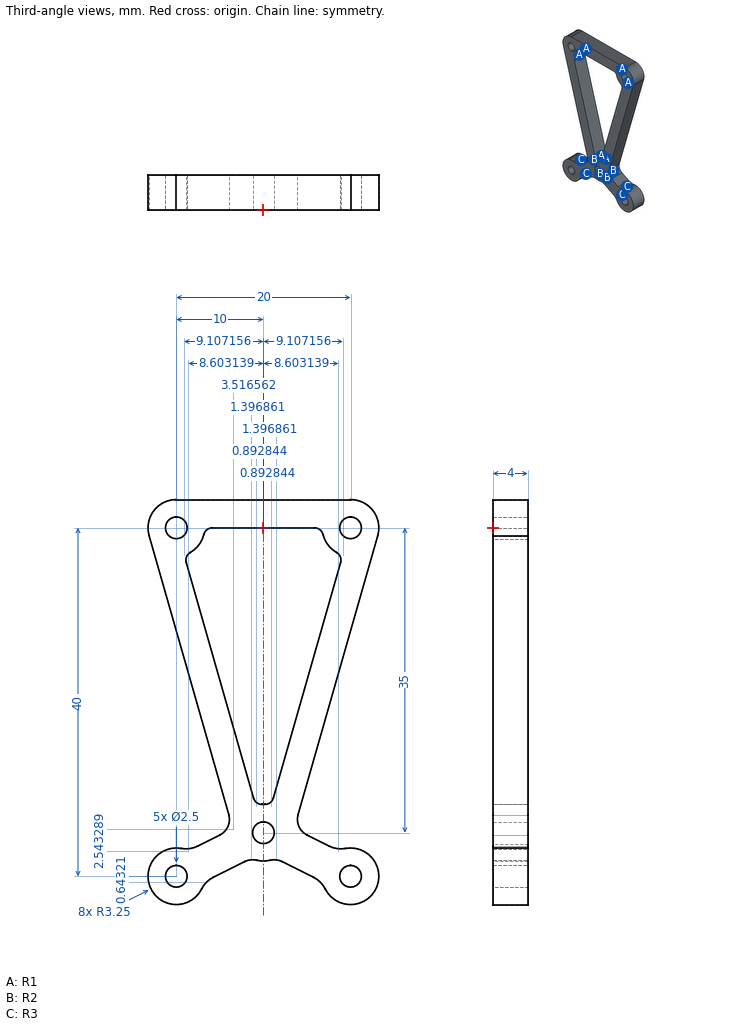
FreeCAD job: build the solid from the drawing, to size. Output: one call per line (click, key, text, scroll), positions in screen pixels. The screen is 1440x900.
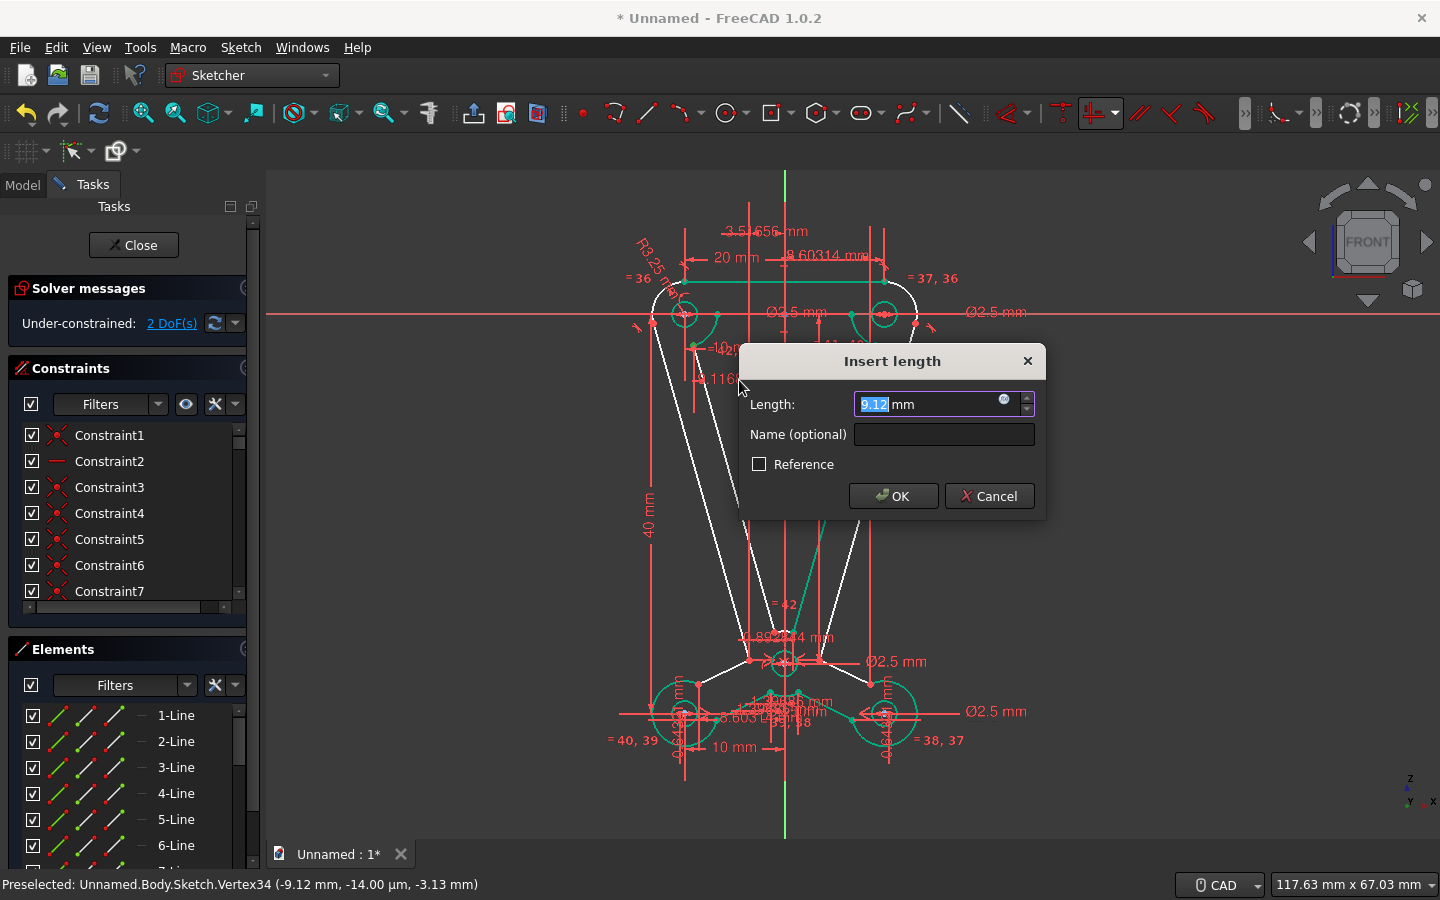
text(9.107156)
key(Return)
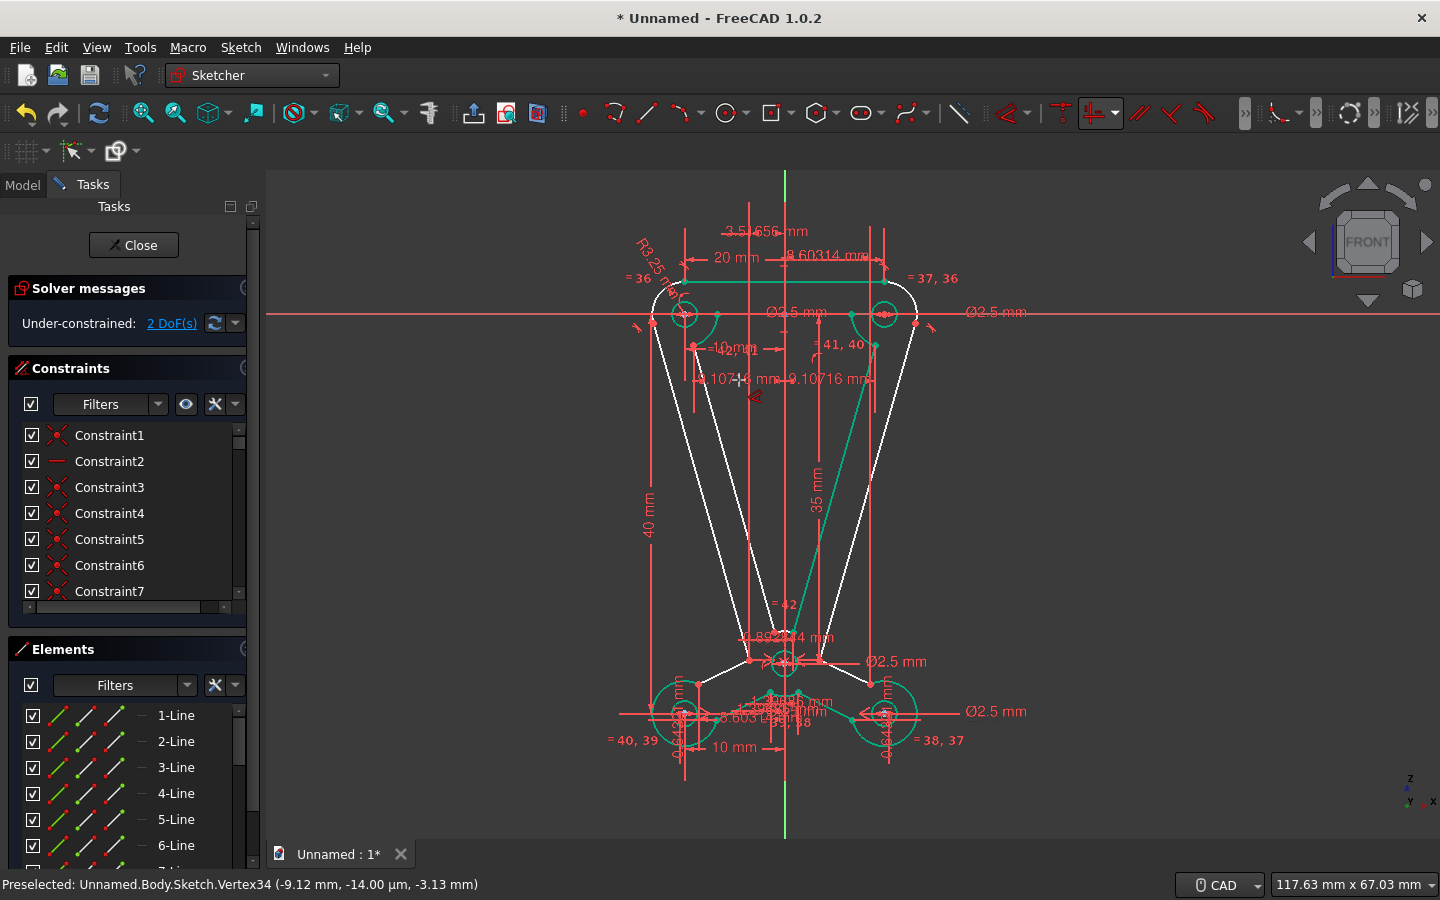
scroll(775, 633, up, 8)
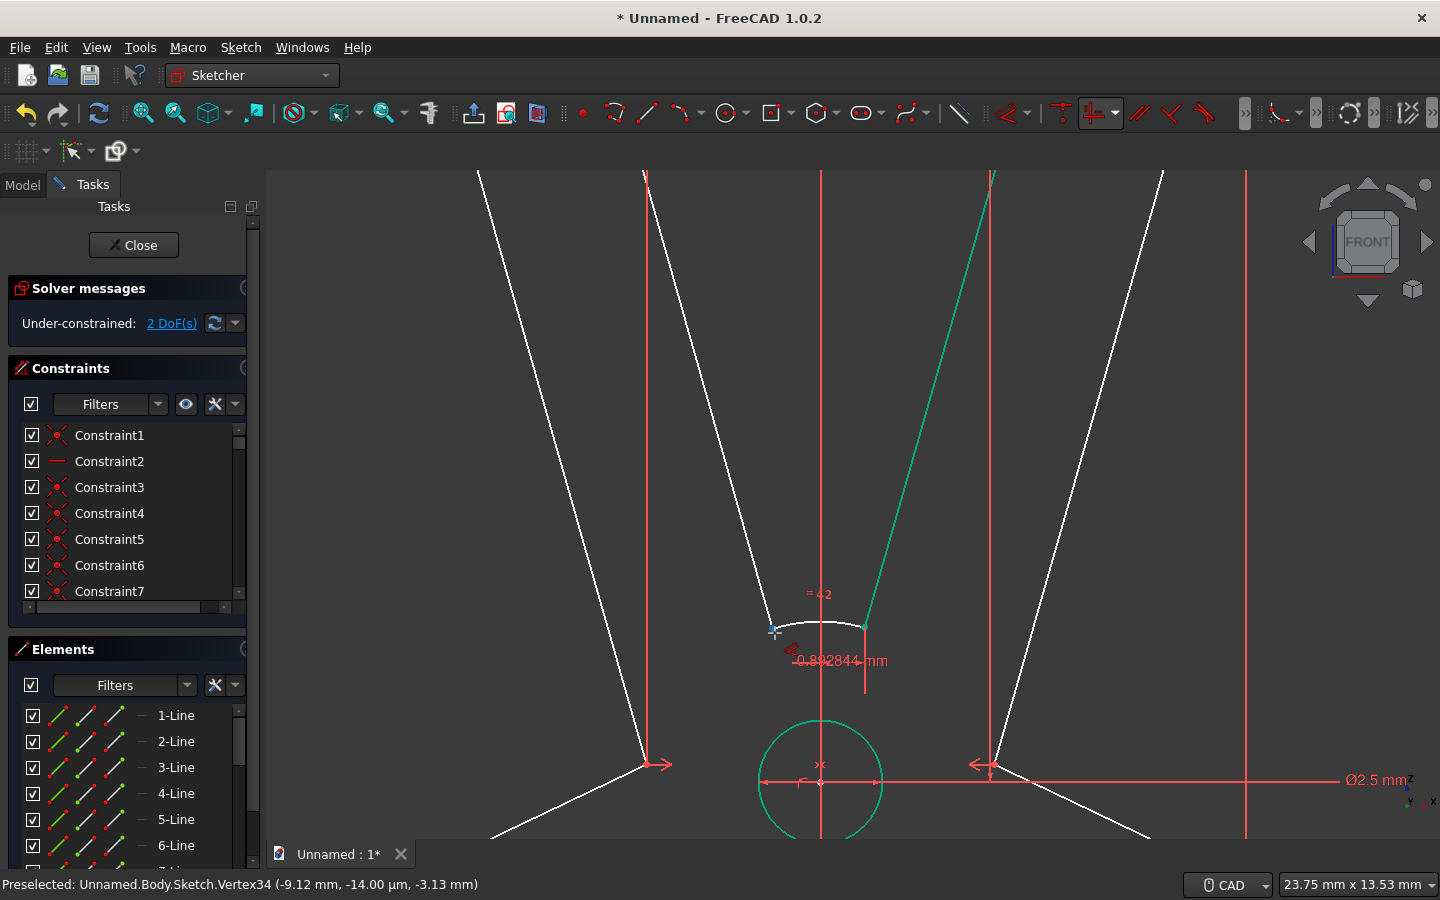
click(773, 629)
click(797, 687)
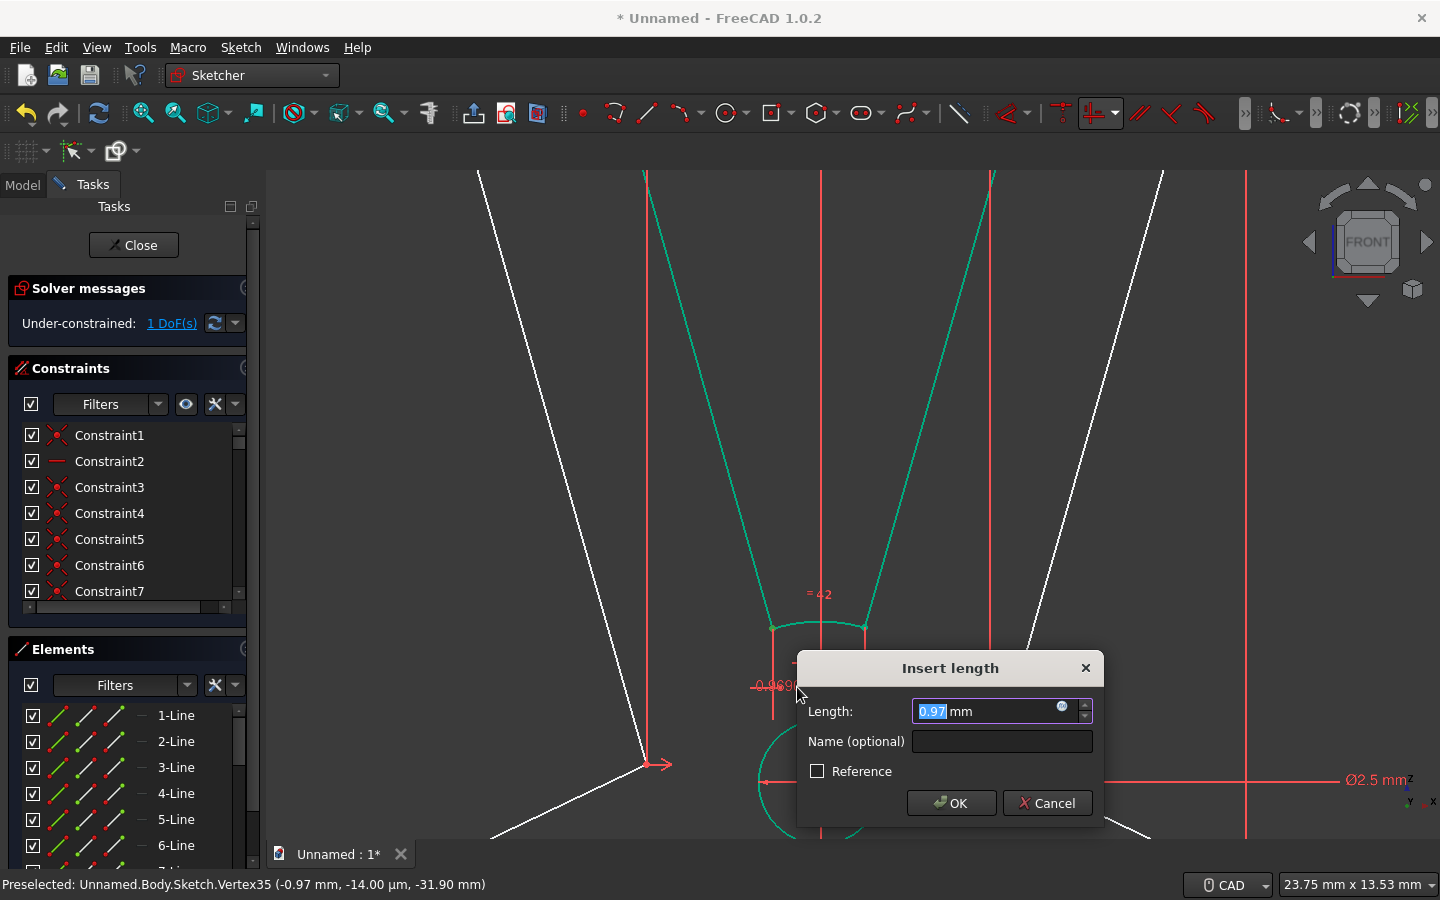
text(0.892844)
key(Return)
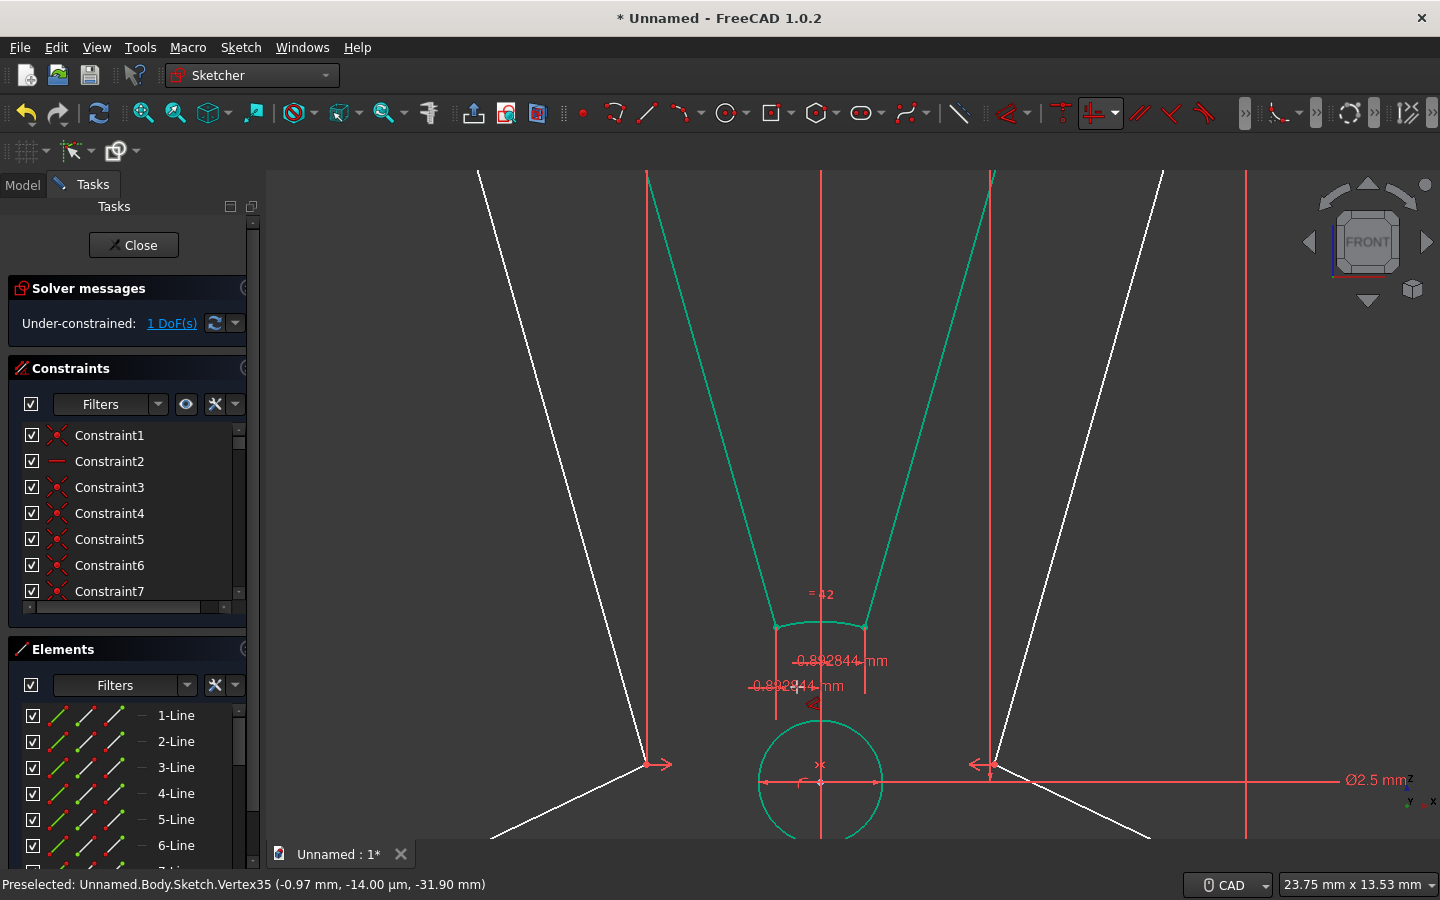
scroll(775, 633, down, 8)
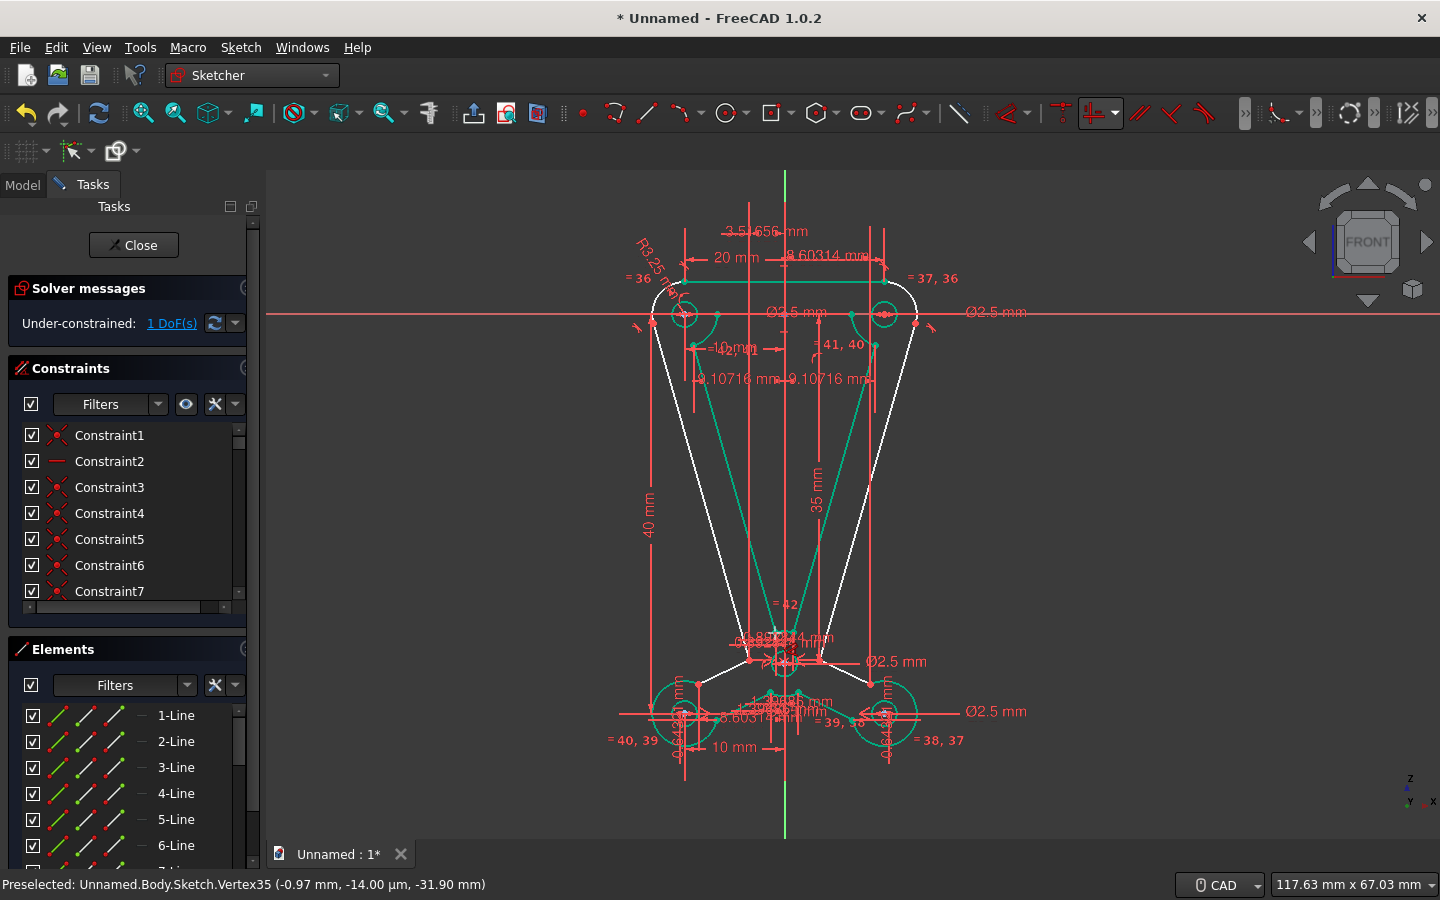
scroll(734, 667, up, 3)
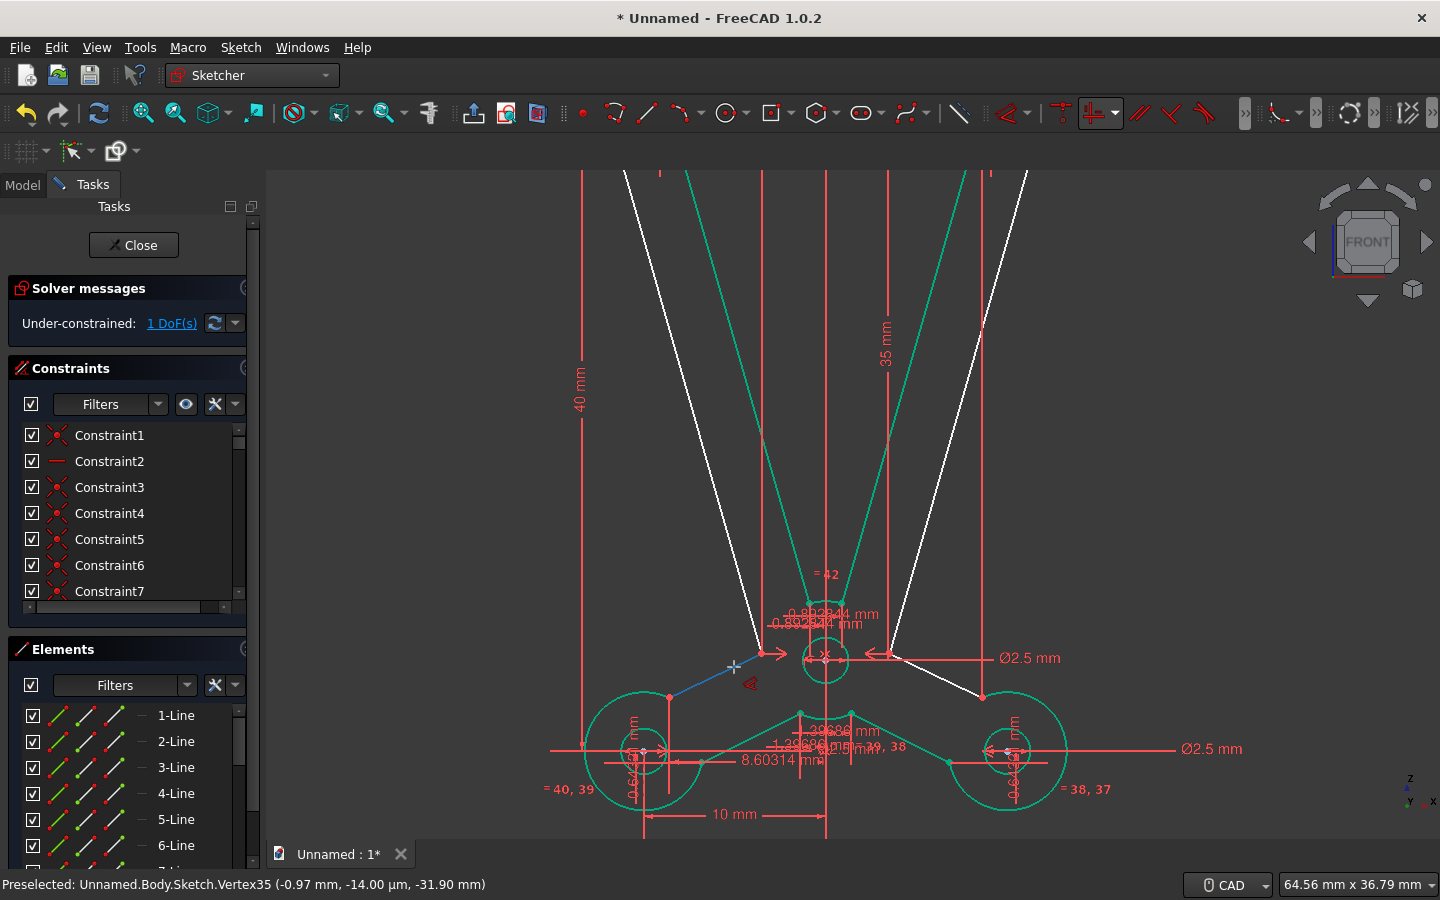
click(734, 667)
click(635, 676)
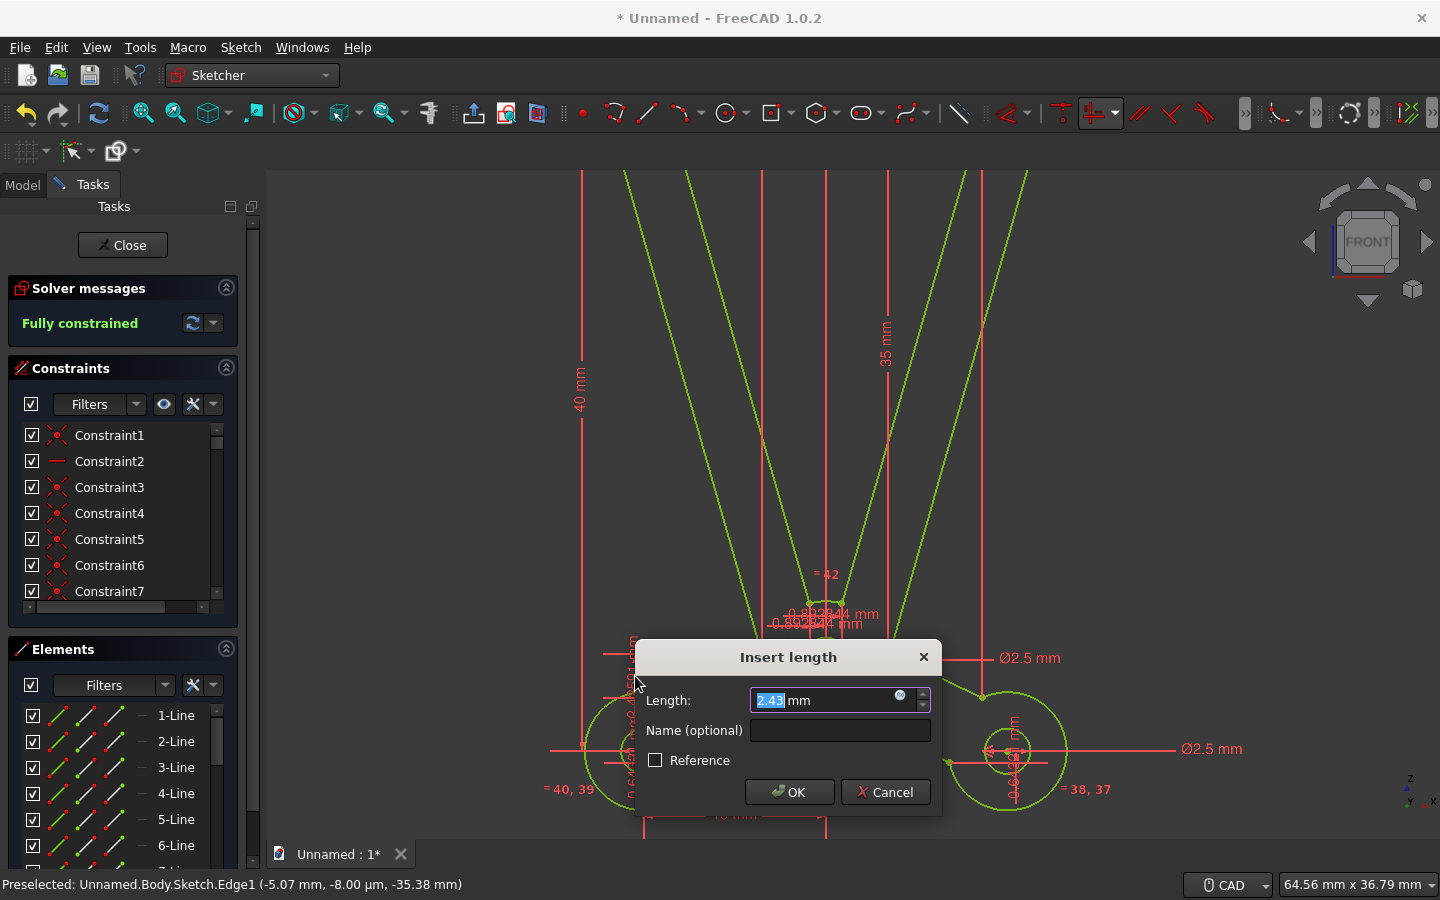
text(2.543289)
key(Return)
key(Escape)